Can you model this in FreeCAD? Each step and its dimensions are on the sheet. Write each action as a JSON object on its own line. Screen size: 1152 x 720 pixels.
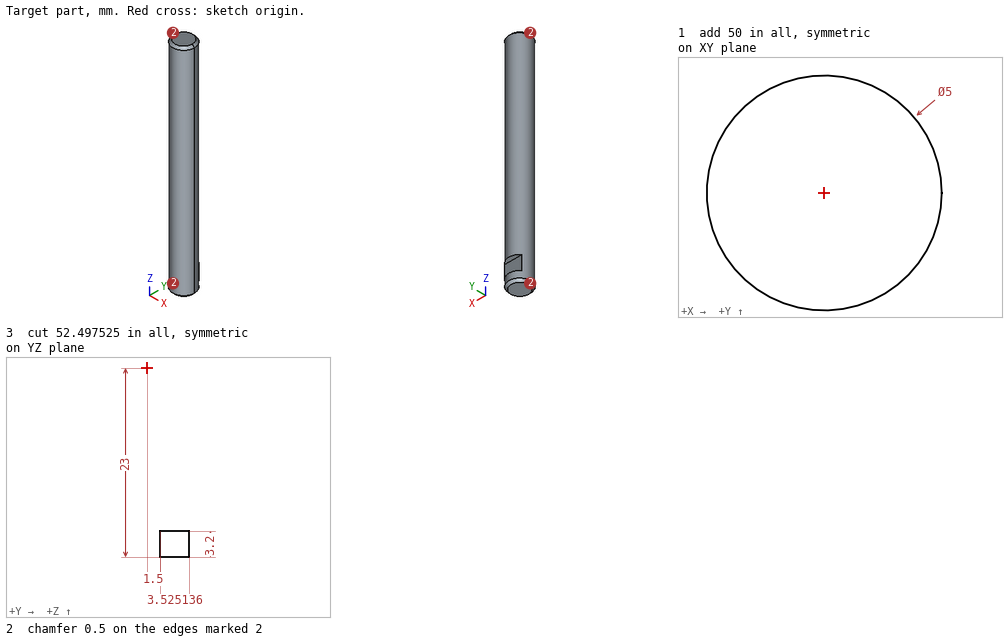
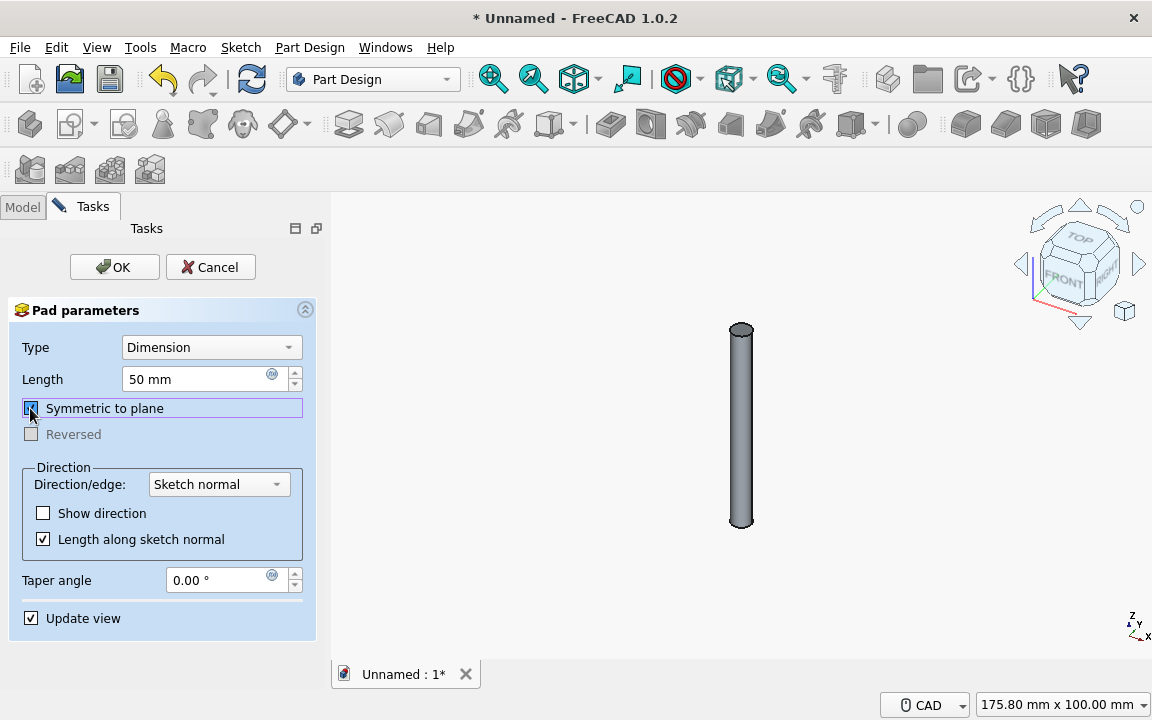
{"action": "left_click", "coordinate": [115, 267]}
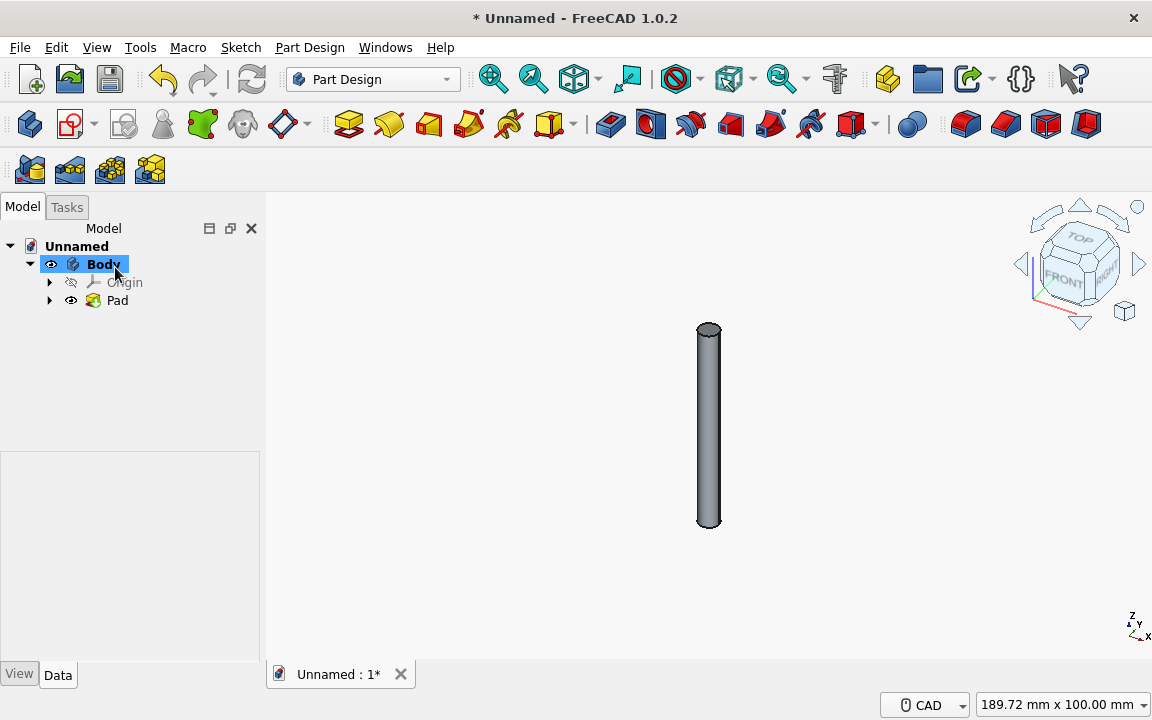
{"action": "key", "text": "v f"}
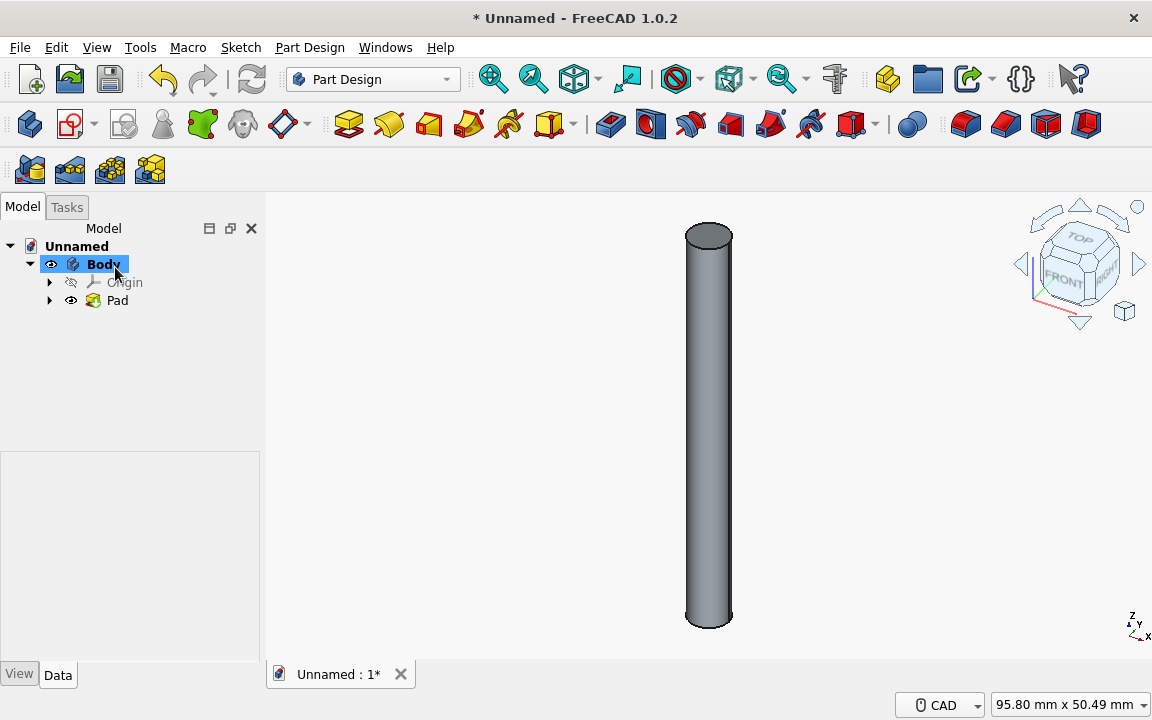
{"action": "left_click", "coordinate": [716, 627]}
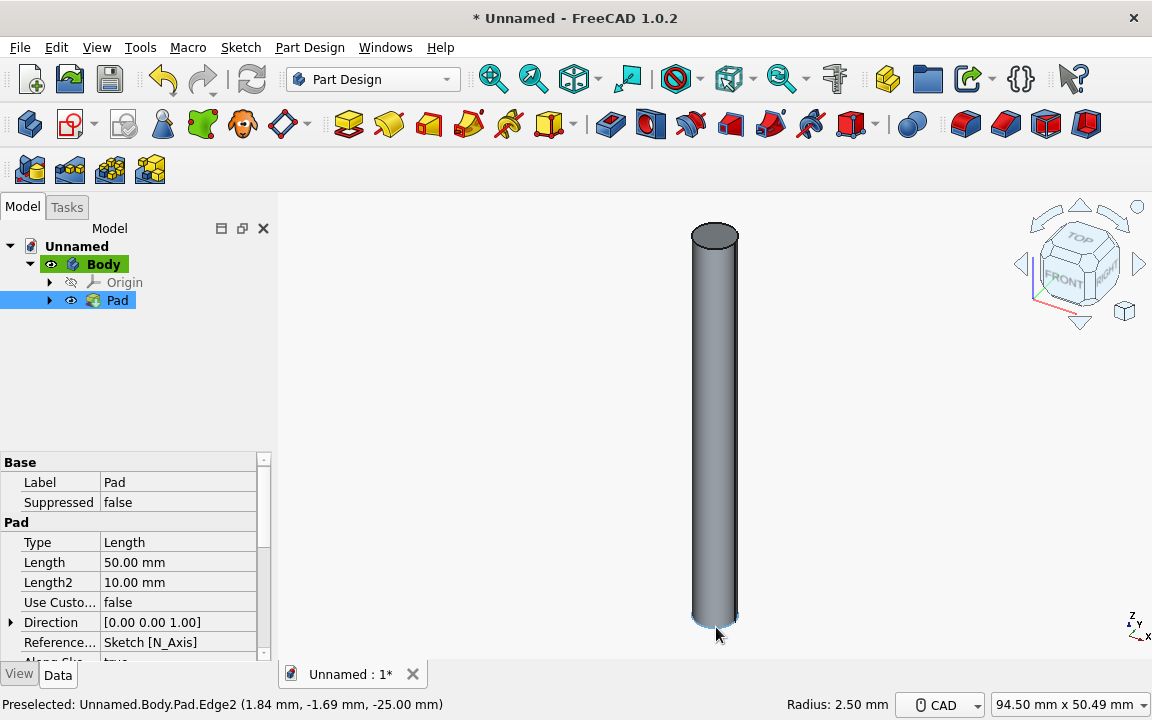
{"action": "left_click", "coordinate": [692, 236], "text": "ctrl"}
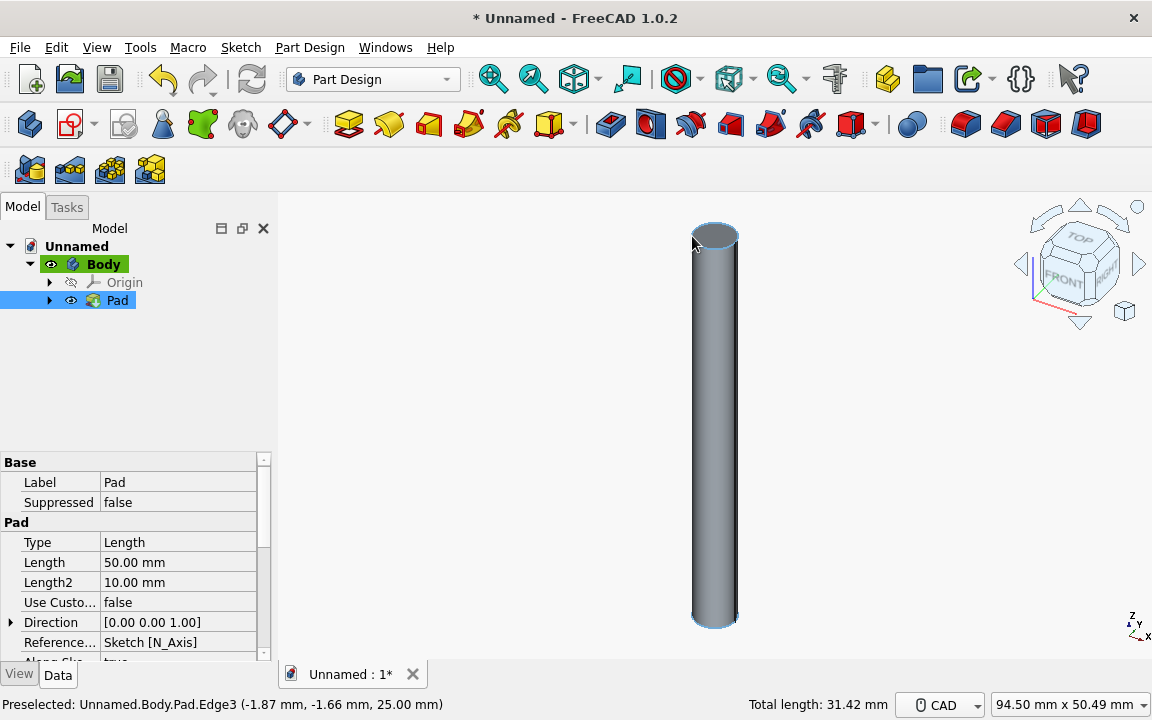
{"action": "left_click", "coordinate": [1006, 124]}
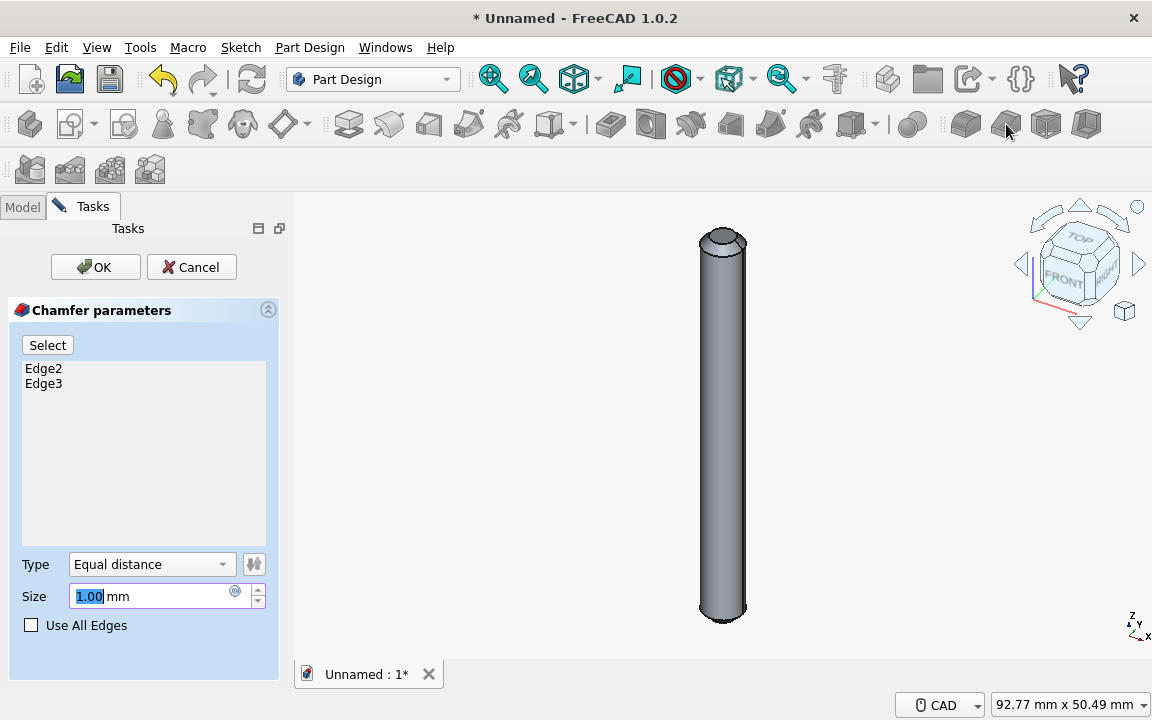
{"action": "type", "text": "0.5"}
{"action": "key", "text": "Tab"}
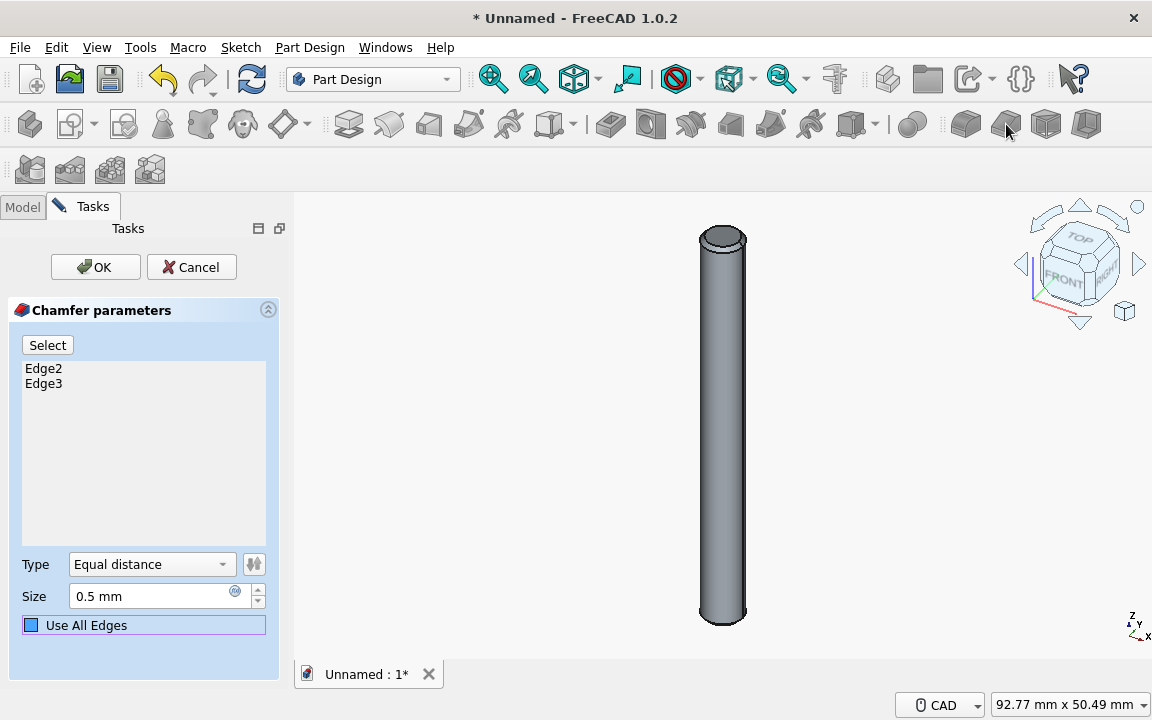
{"action": "left_click", "coordinate": [96, 267]}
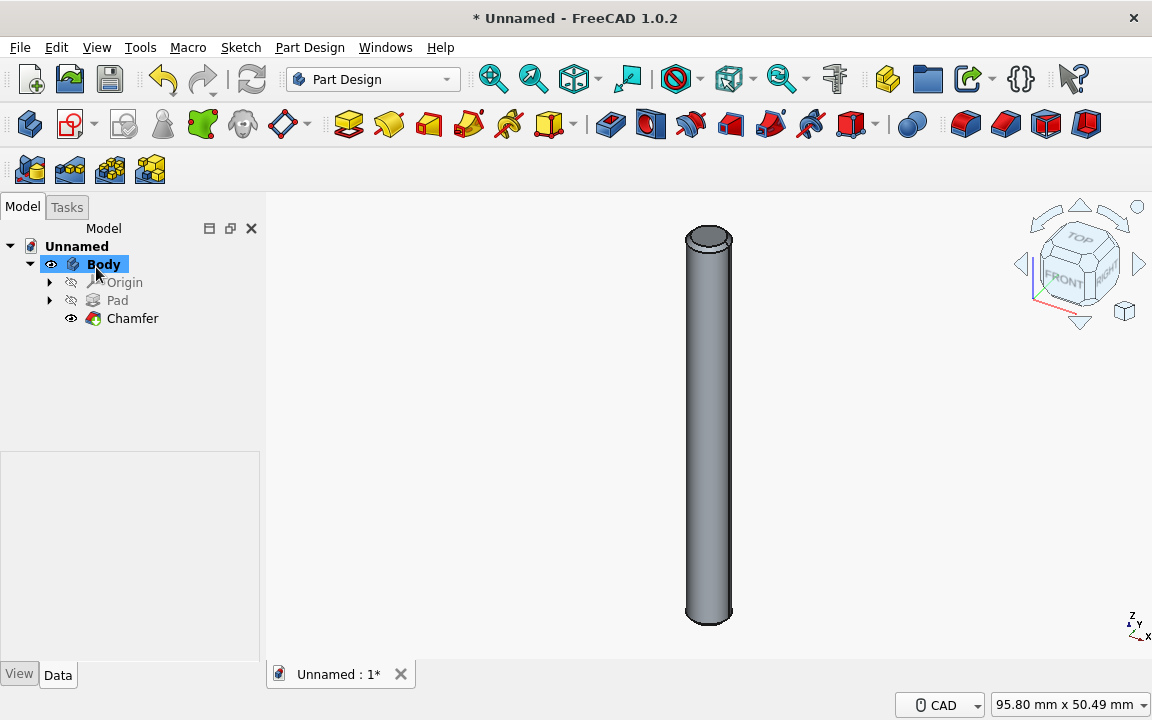
{"action": "left_click", "coordinate": [70, 124]}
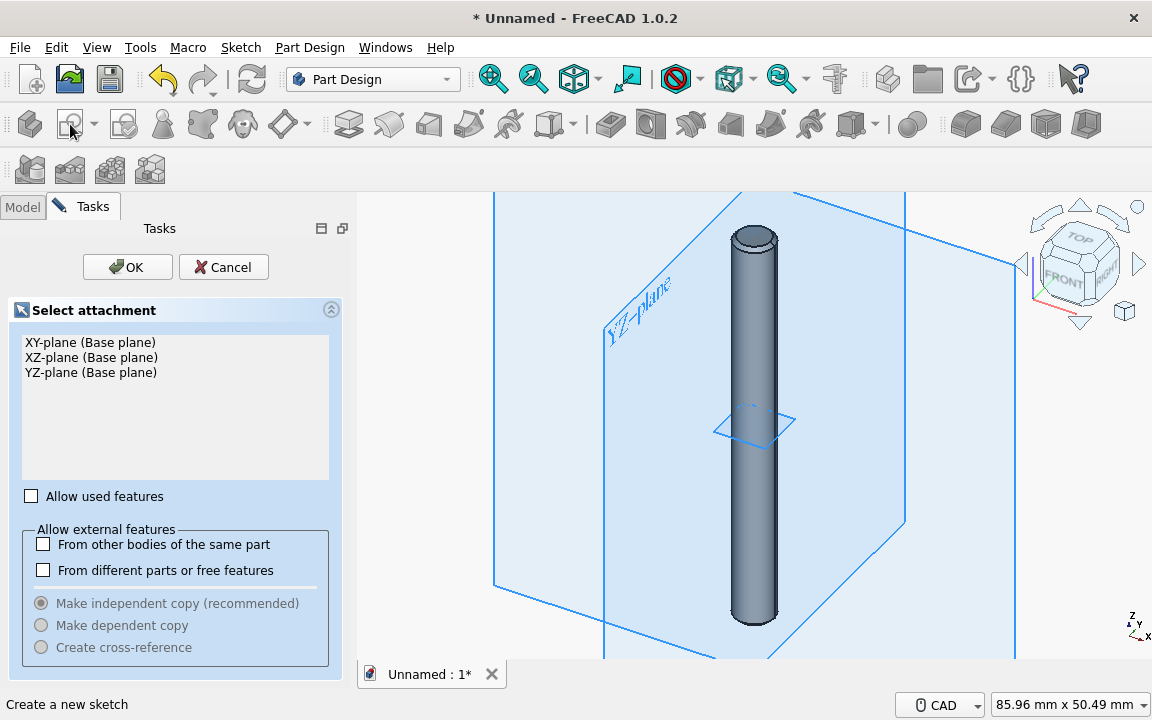
{"action": "left_click", "coordinate": [82, 372]}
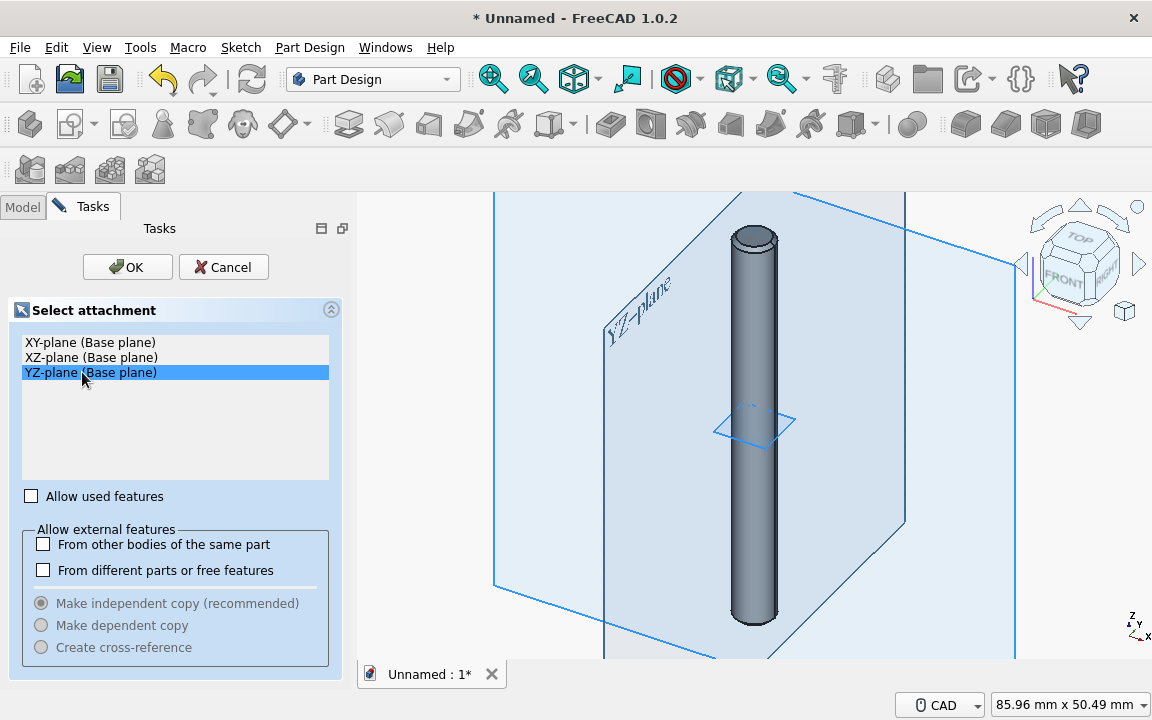
{"action": "left_click", "coordinate": [128, 267]}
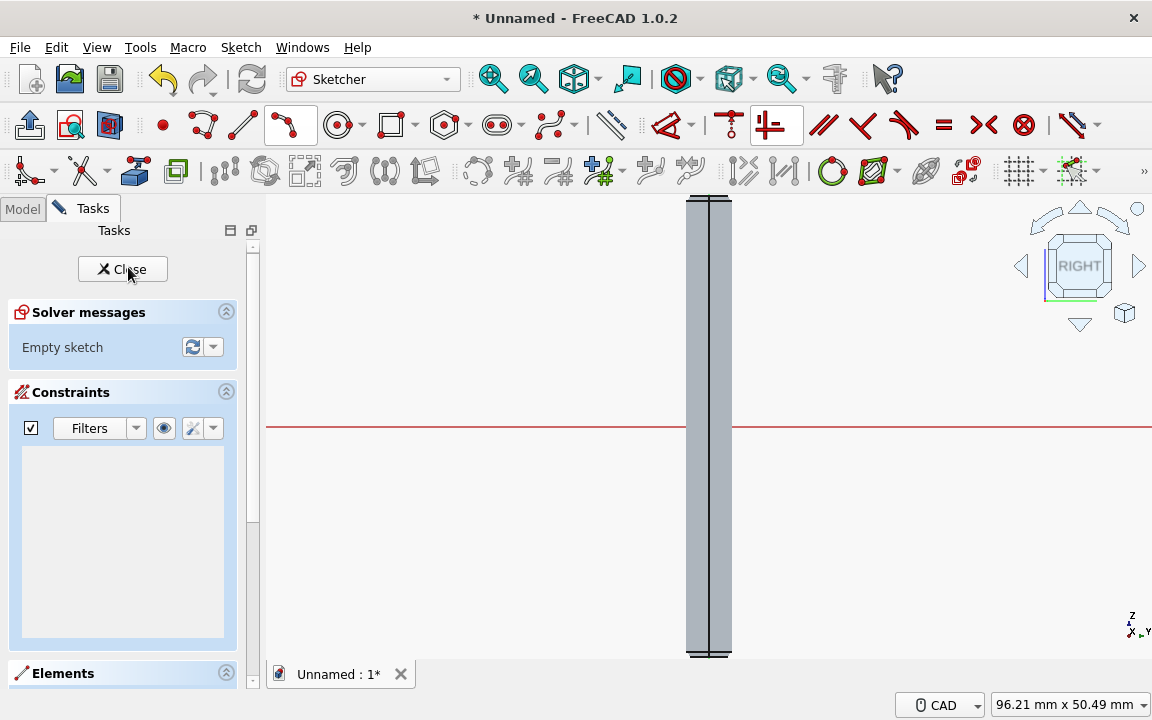
{"action": "left_click", "coordinate": [110, 126]}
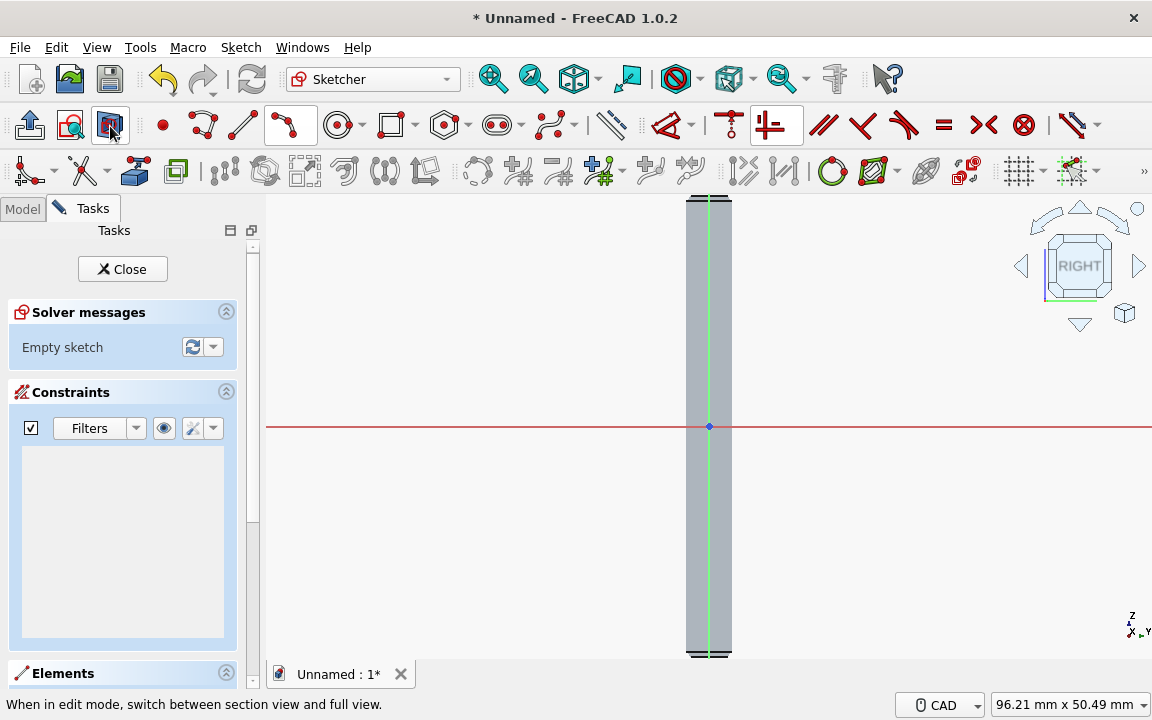
{"action": "scroll", "coordinate": [640, 426], "scroll_direction": "down", "scroll_amount": 5}